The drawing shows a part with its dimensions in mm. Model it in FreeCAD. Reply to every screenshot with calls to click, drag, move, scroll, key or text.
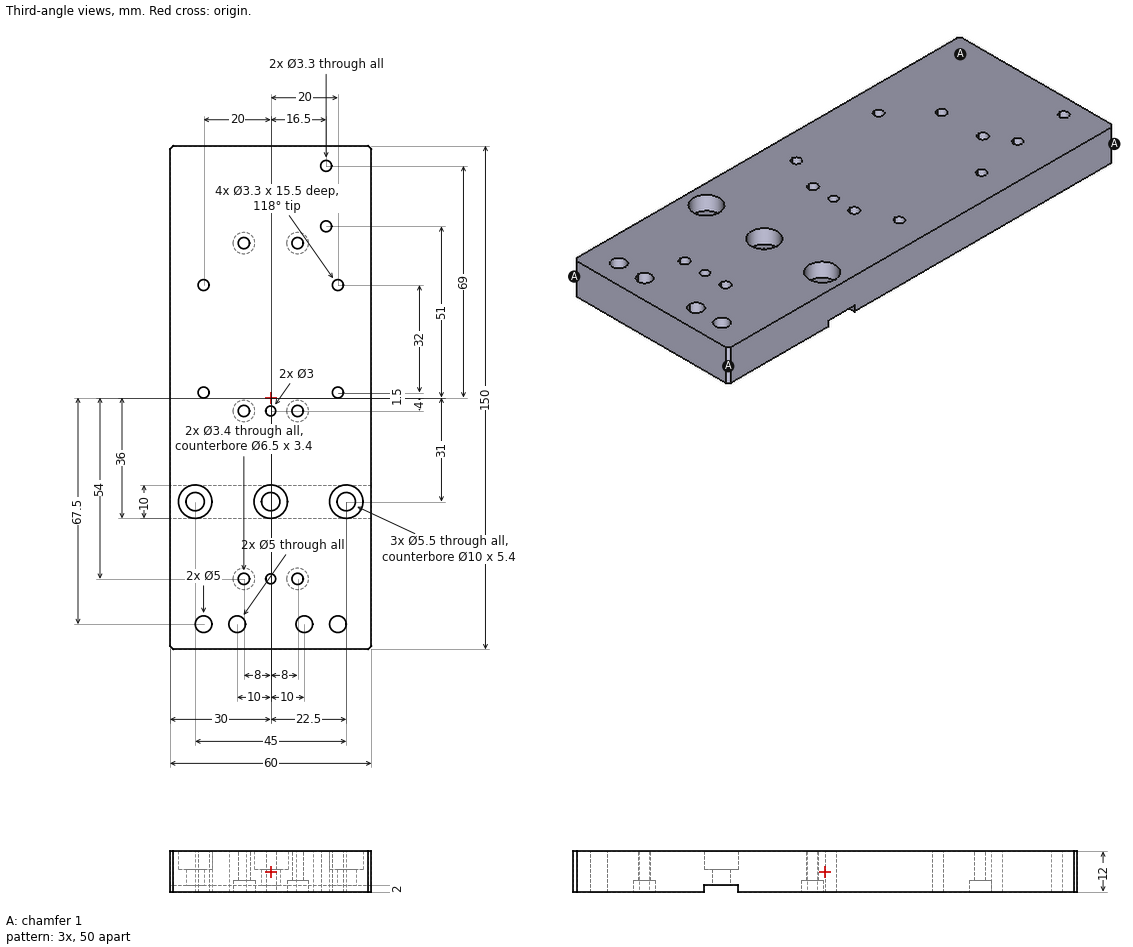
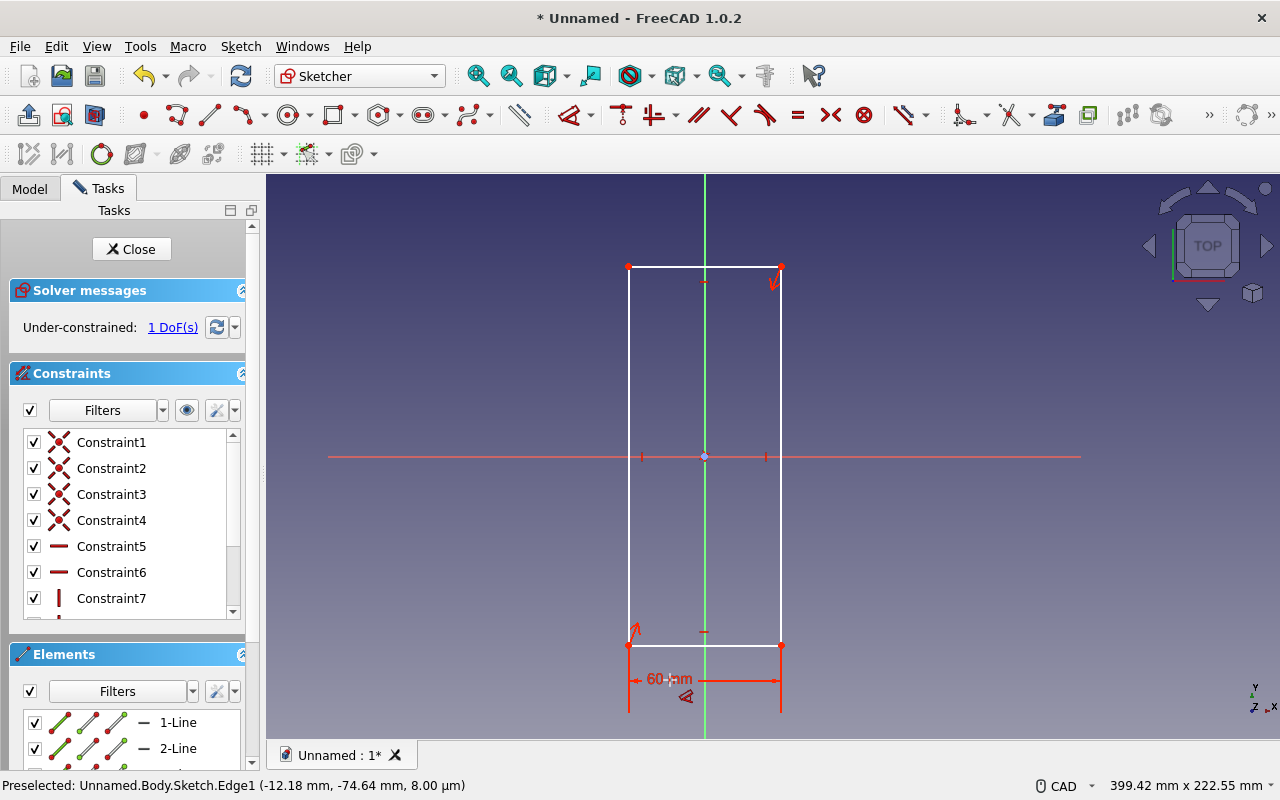
click(781, 532)
click(815, 369)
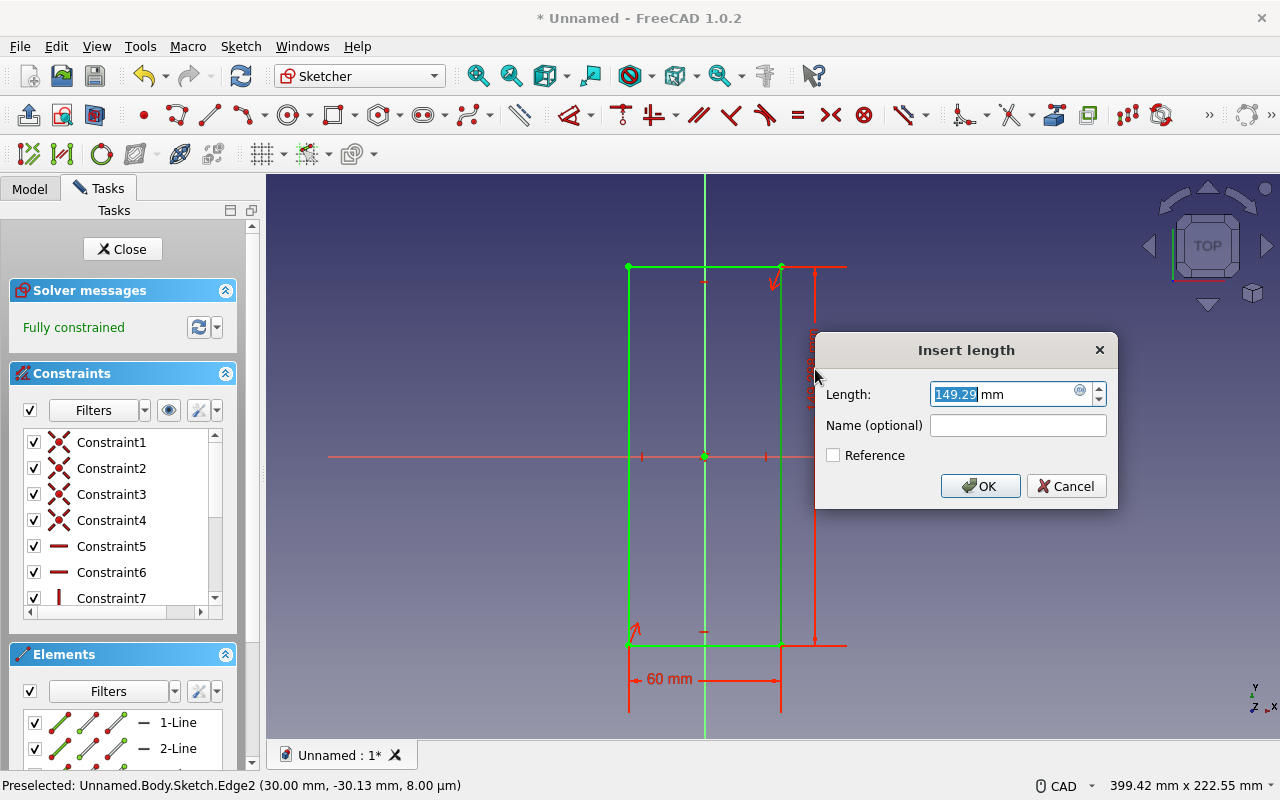
text(150)
key(Return)
key(Escape)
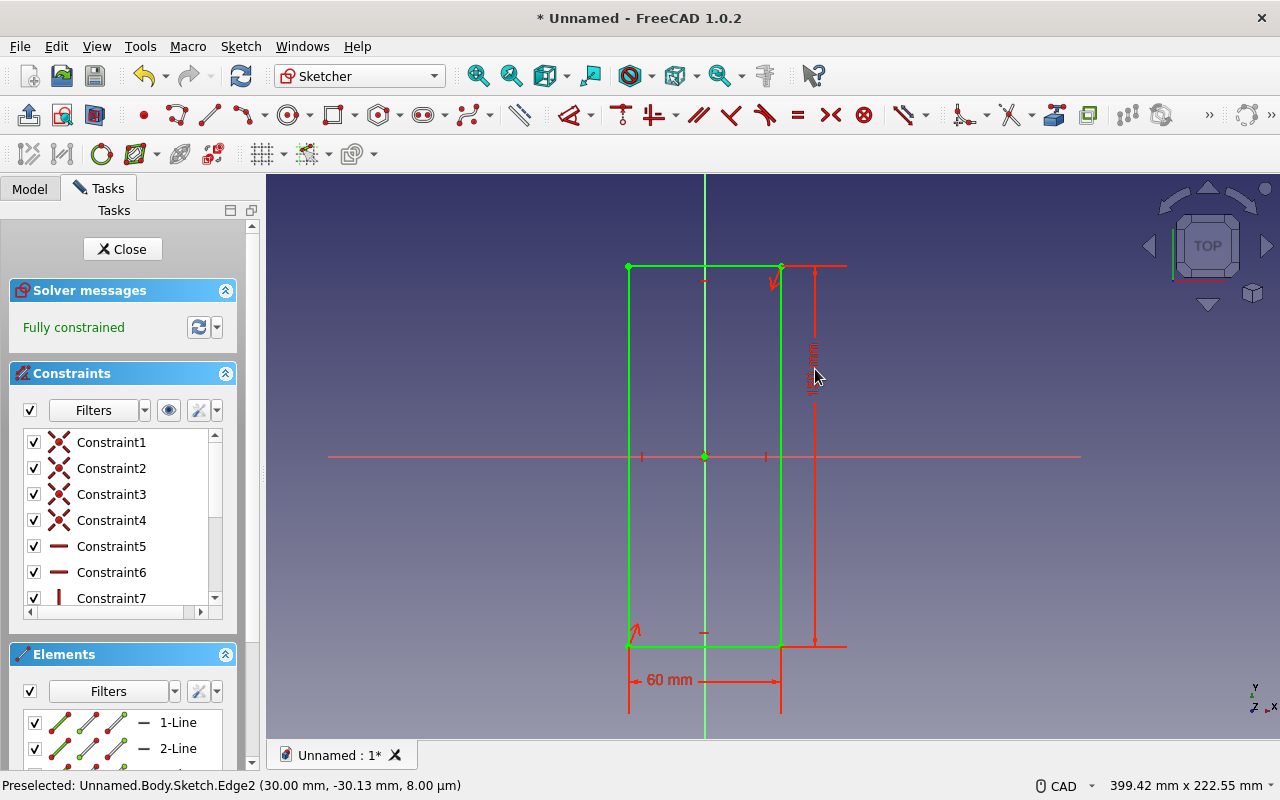
click(123, 249)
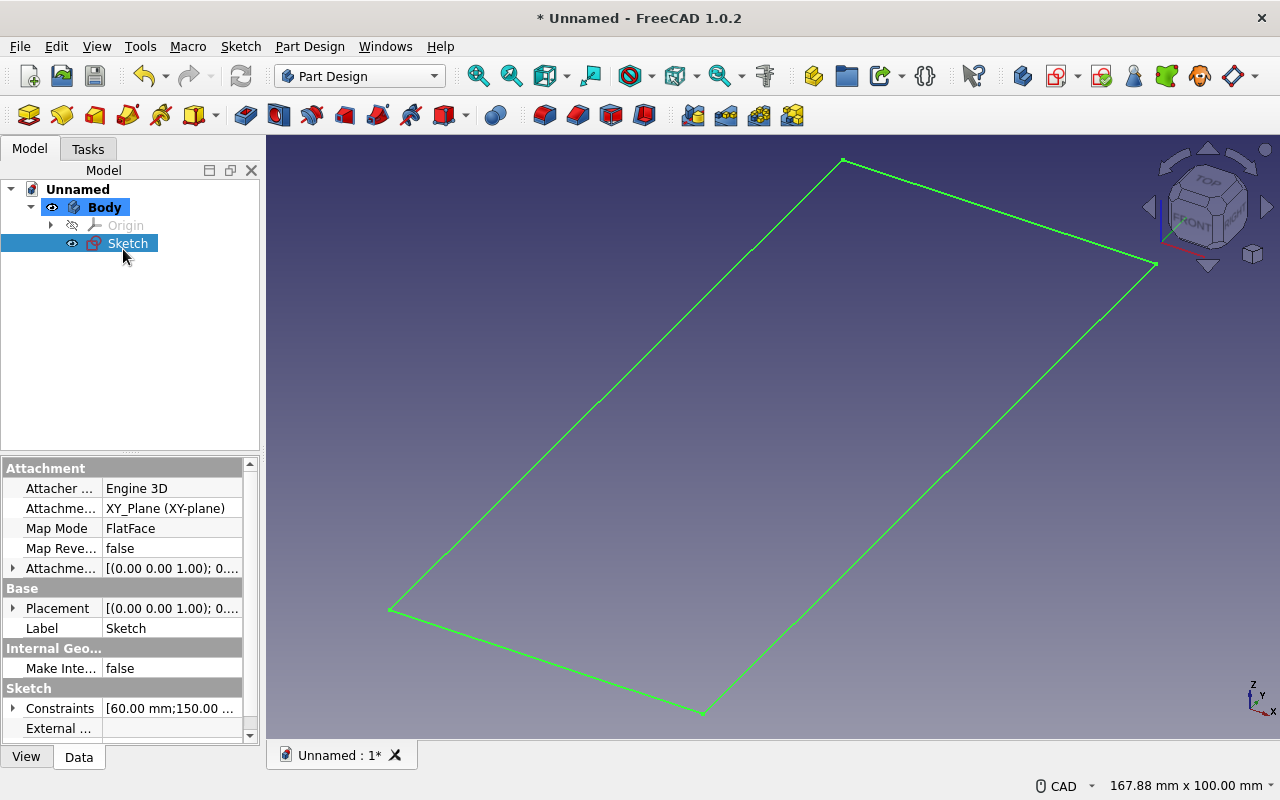
click(29, 116)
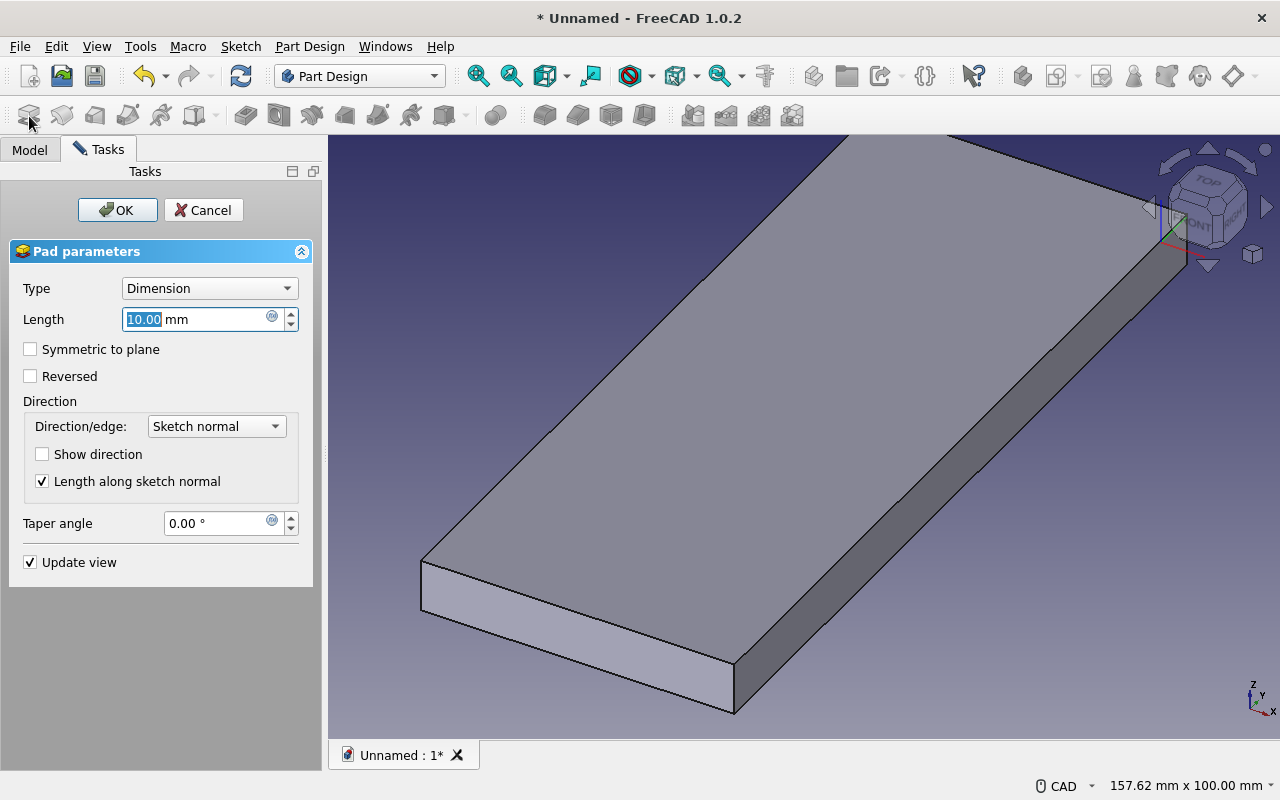
text(12)
key(Tab)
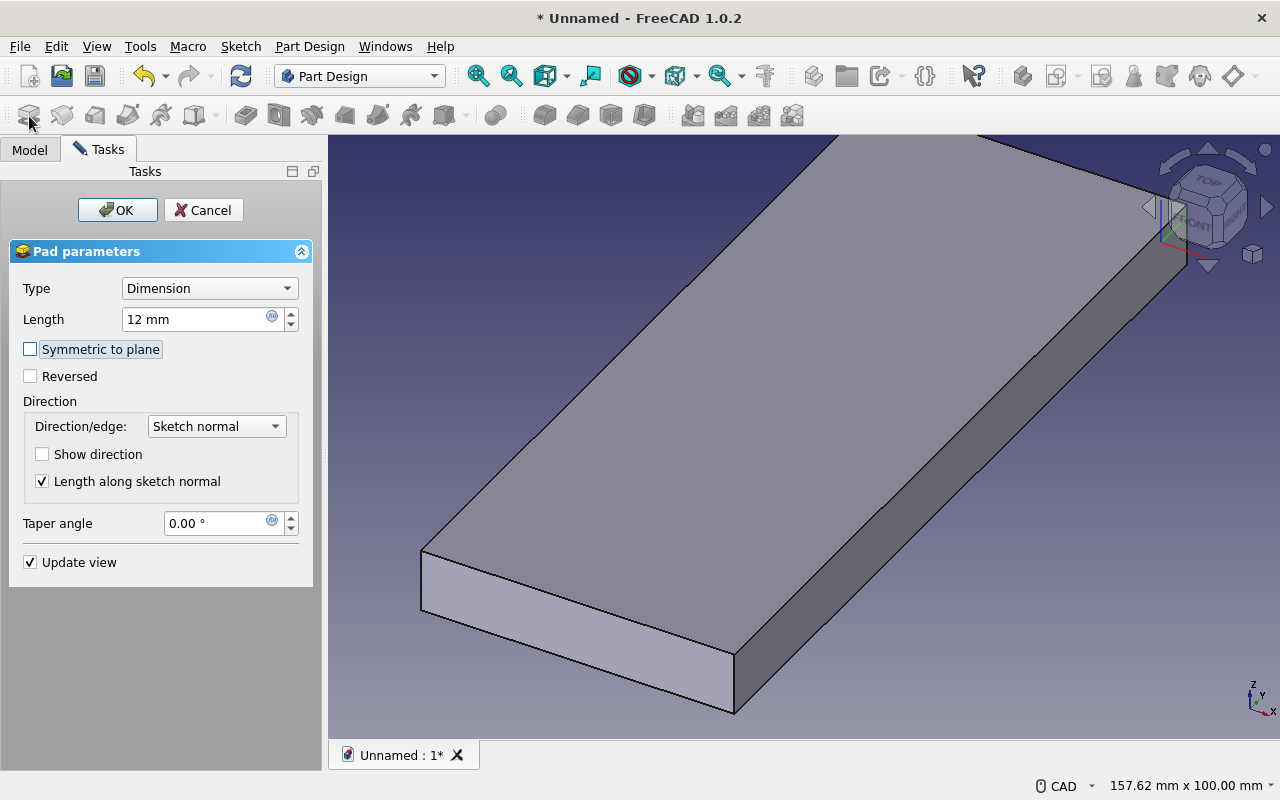
click(31, 349)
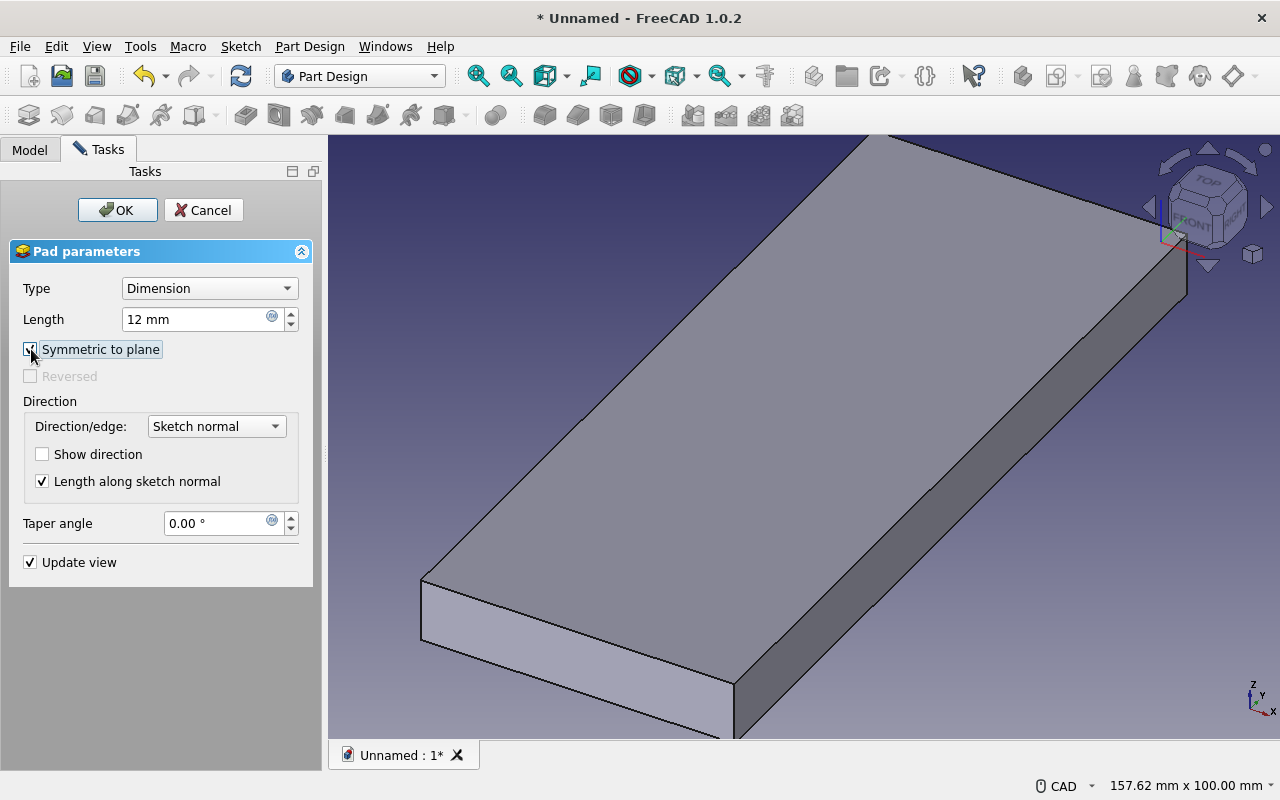
click(118, 210)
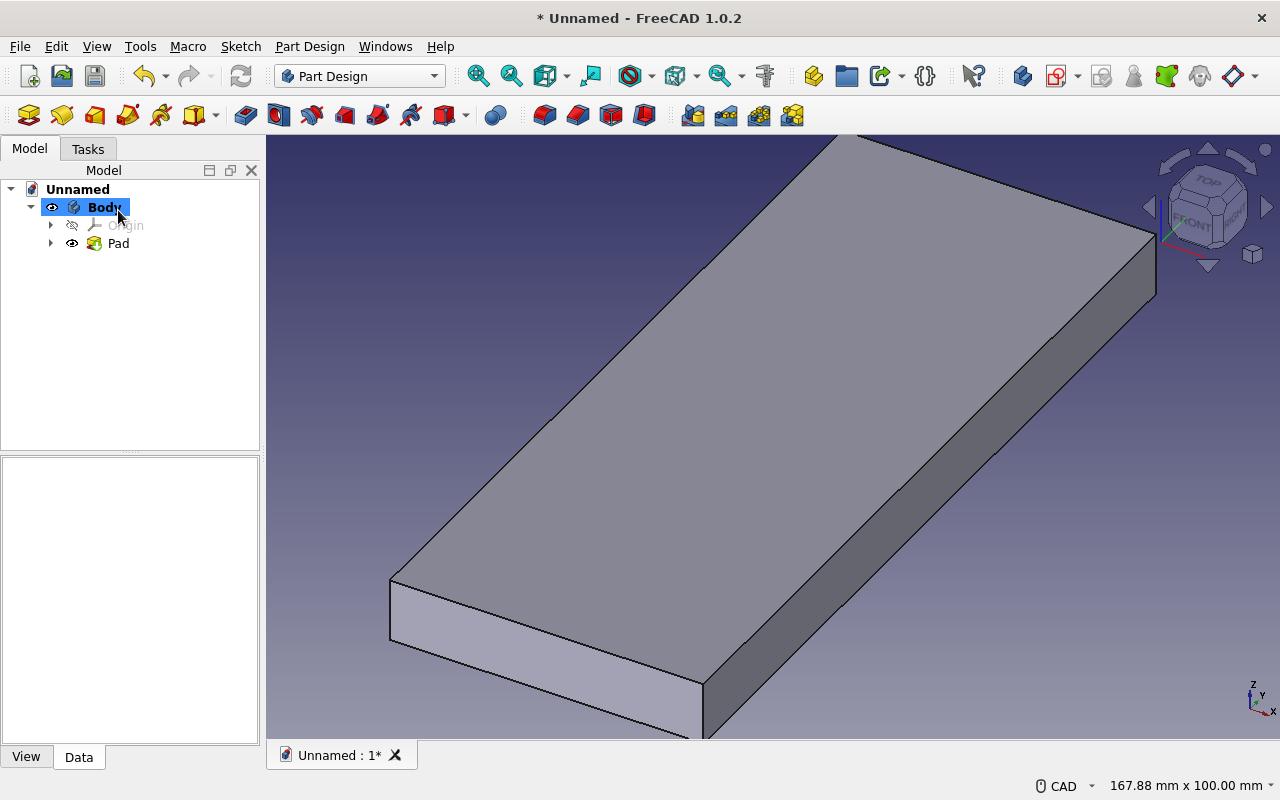
click(479, 76)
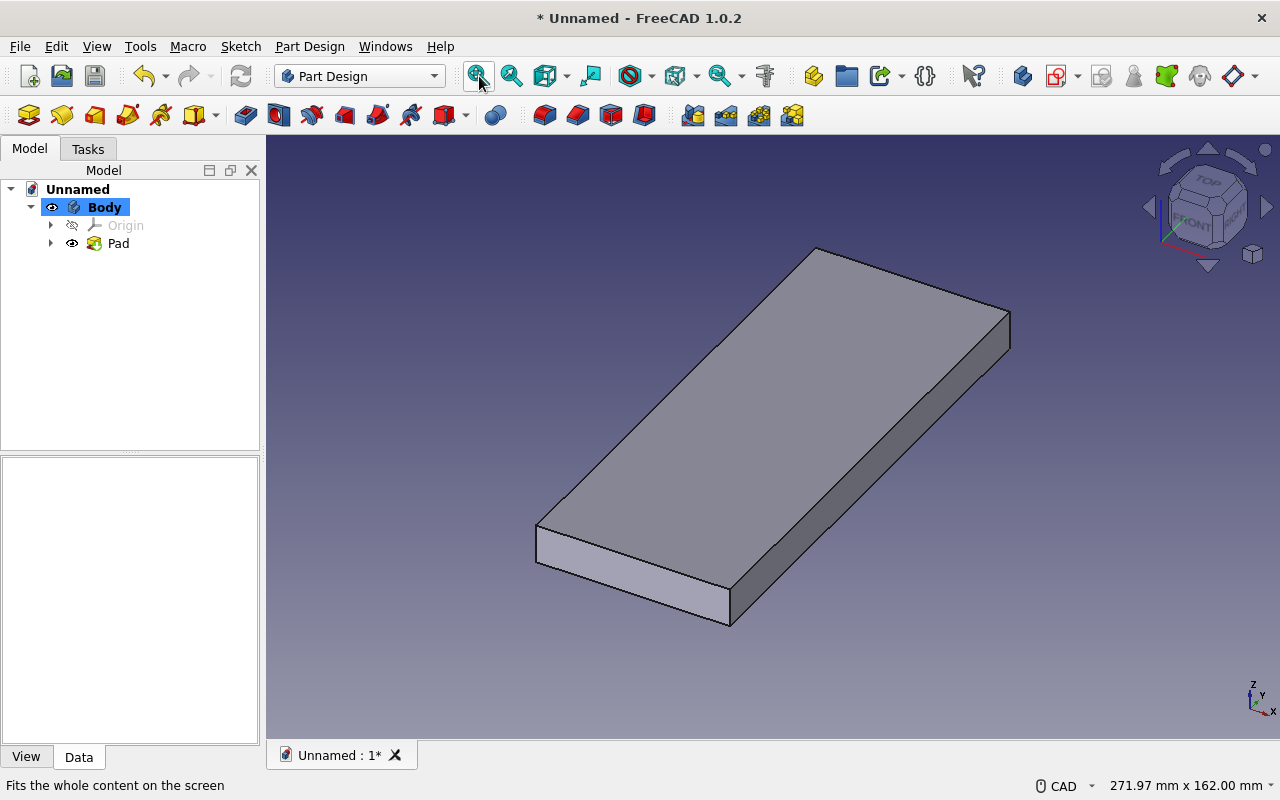
key(5)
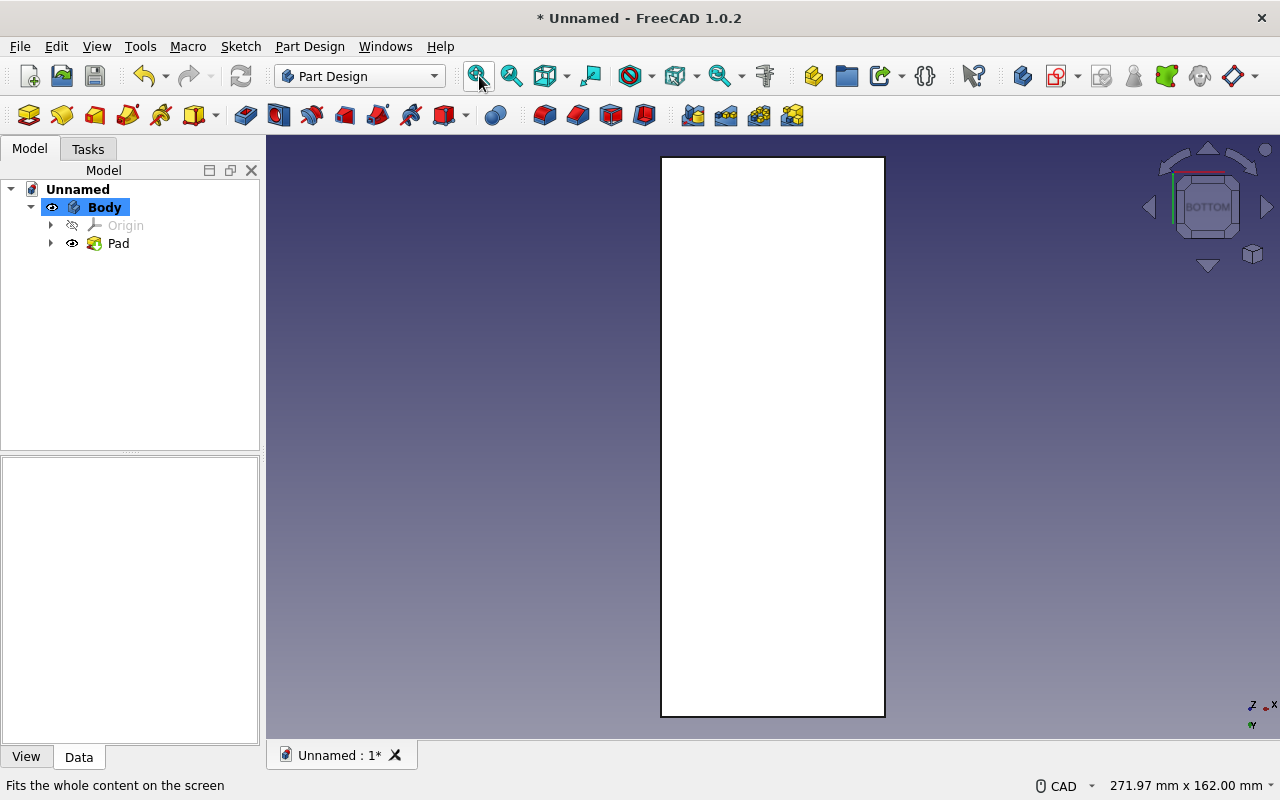
click(773, 596)